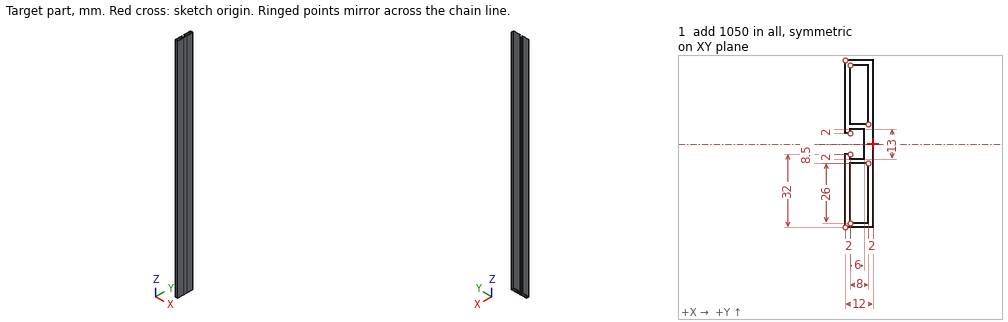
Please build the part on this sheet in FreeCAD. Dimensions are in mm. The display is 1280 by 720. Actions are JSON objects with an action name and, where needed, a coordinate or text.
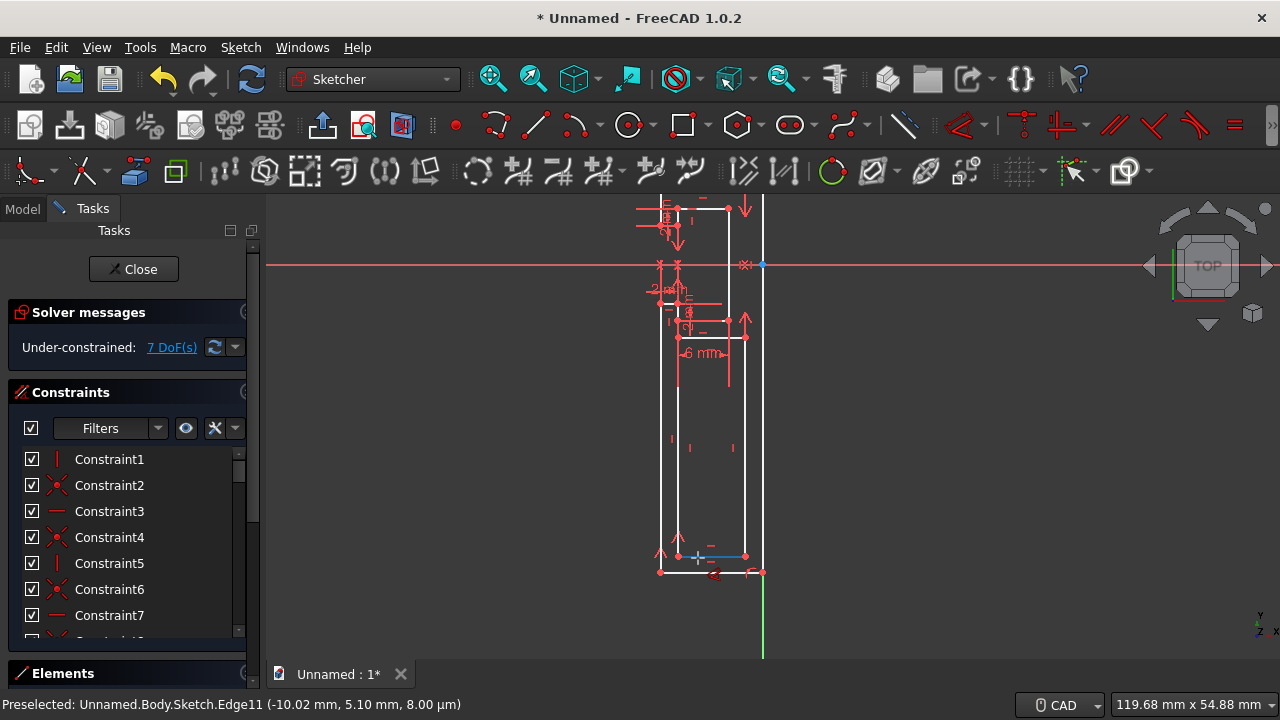
{"action": "left_click", "coordinate": [699, 557]}
{"action": "left_click", "coordinate": [712, 591]}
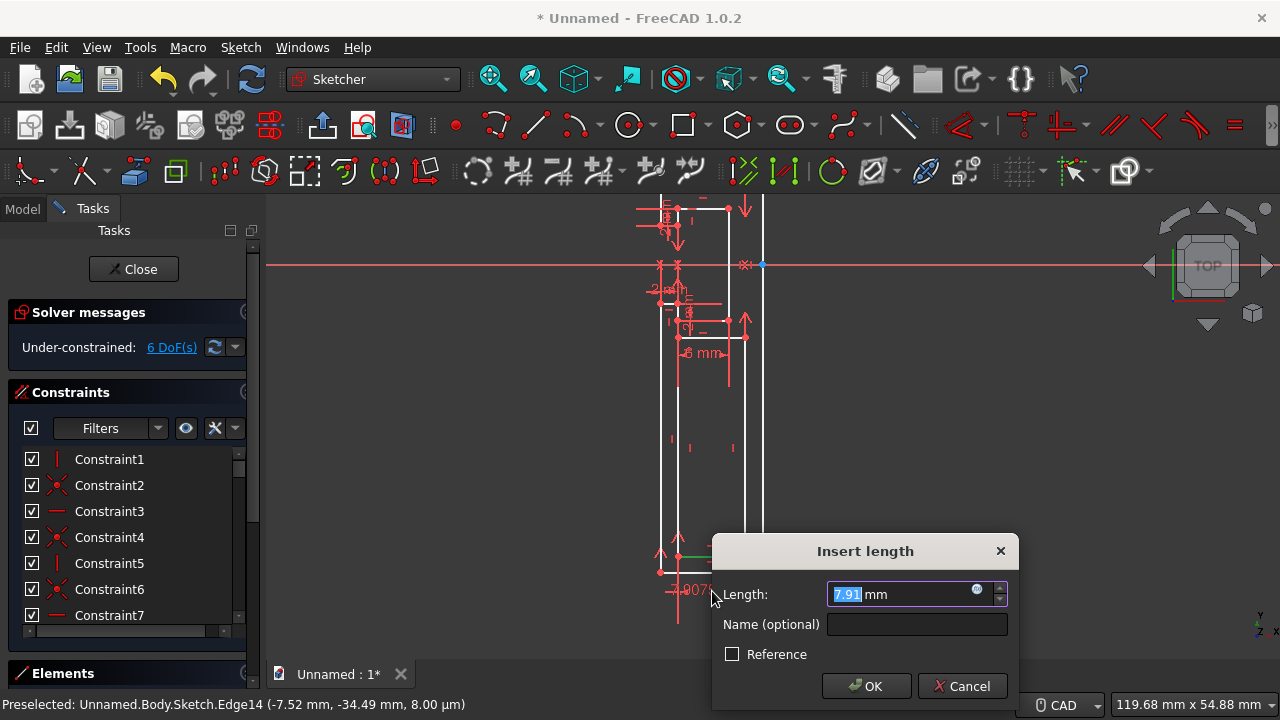
{"action": "type", "text": "8"}
{"action": "key", "text": "Return"}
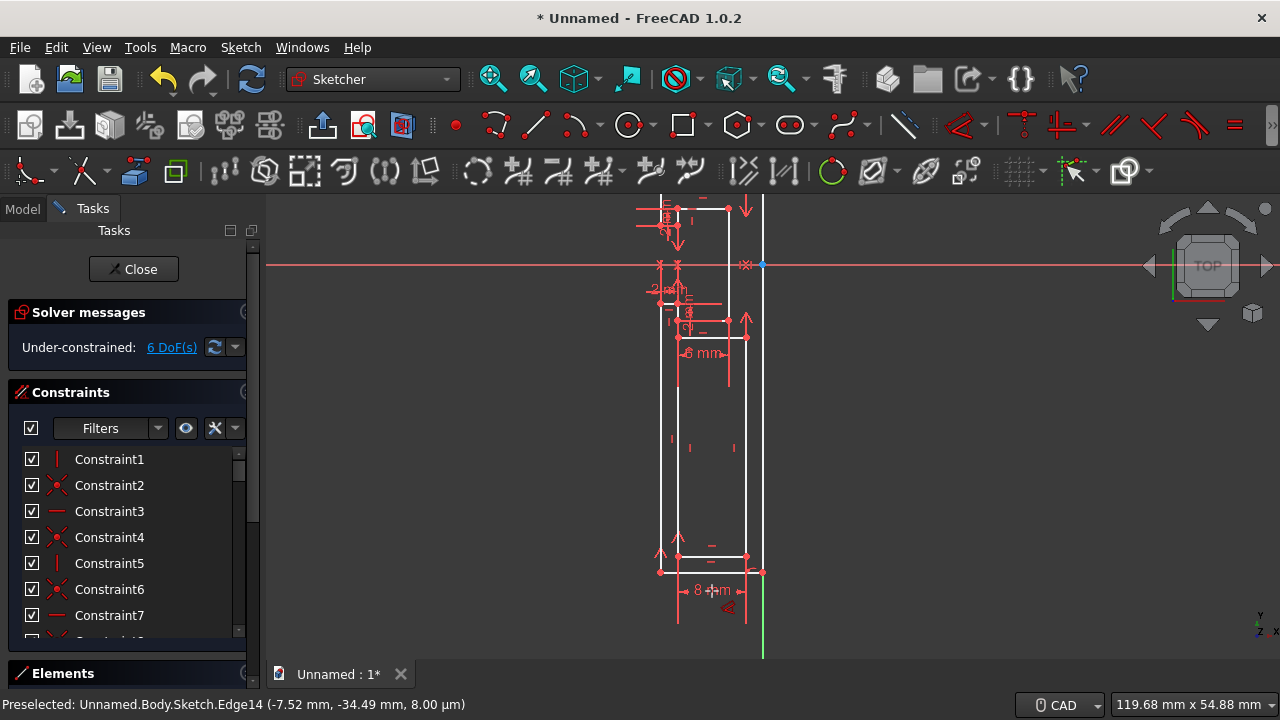
{"action": "left_click", "coordinate": [729, 242]}
{"action": "left_click", "coordinate": [695, 249]}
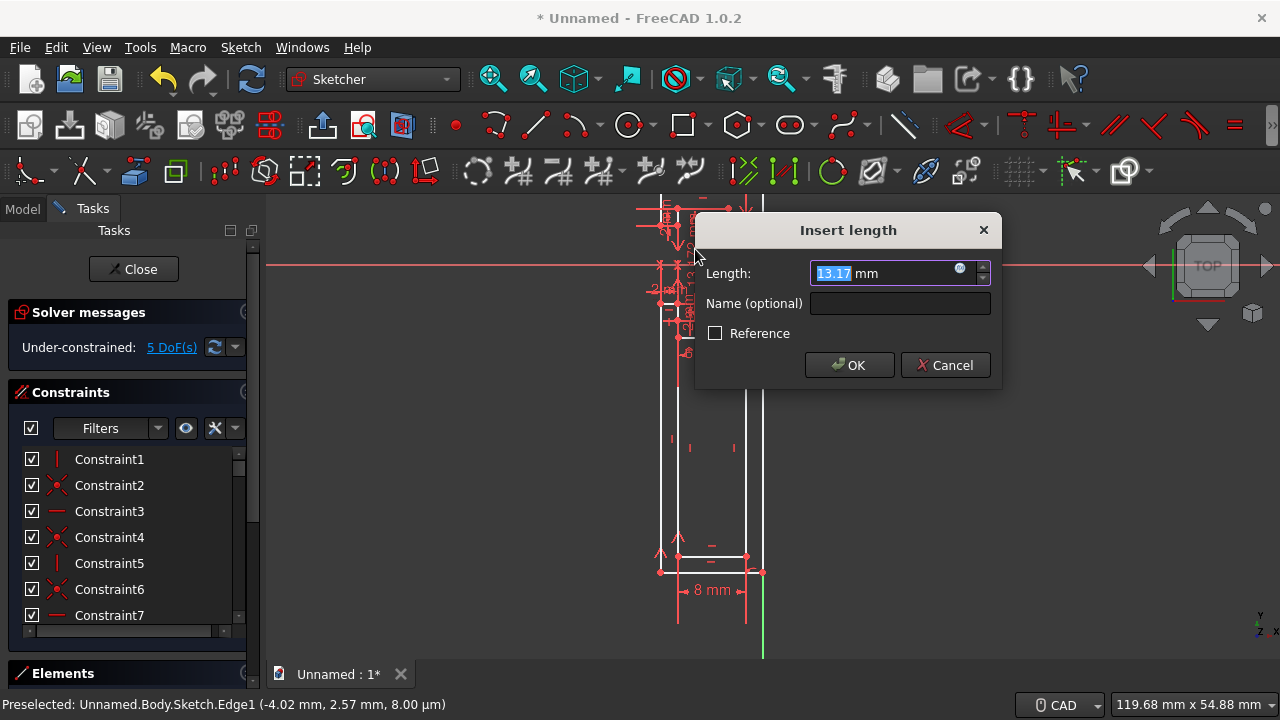
{"action": "type", "text": "13"}
{"action": "key", "text": "Return"}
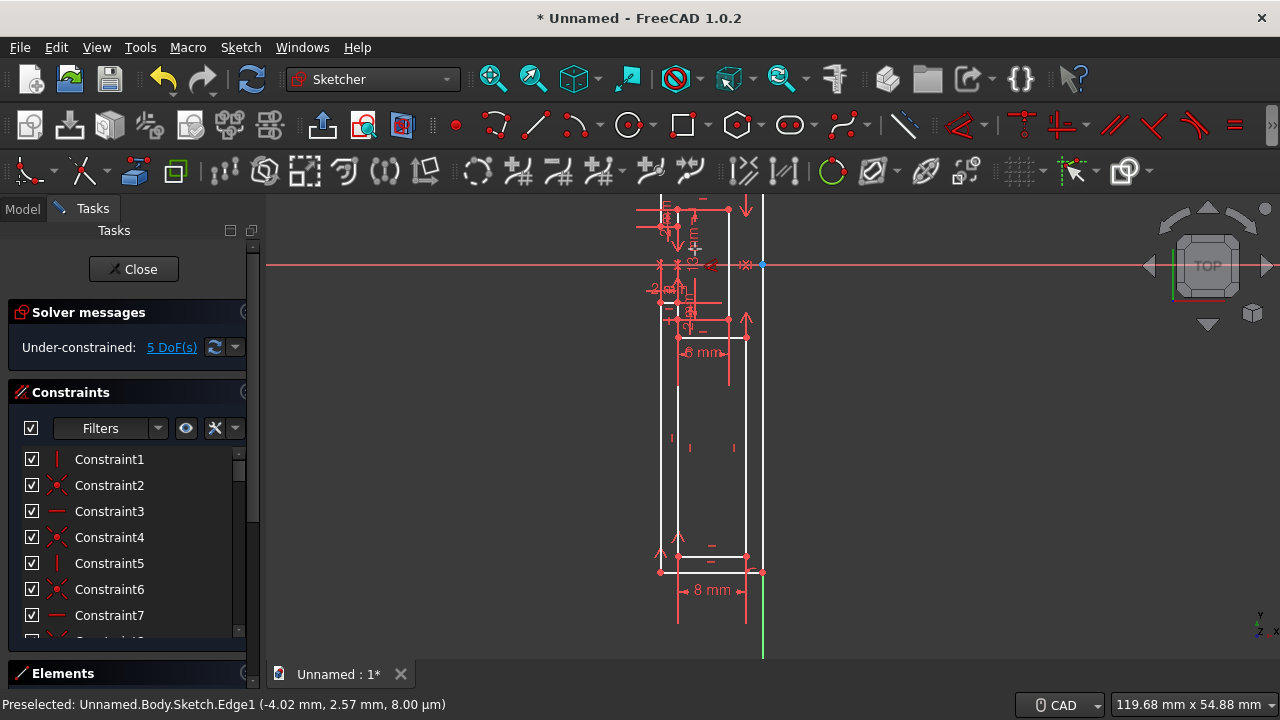
{"action": "left_click", "coordinate": [661, 384]}
{"action": "left_click", "coordinate": [627, 438]}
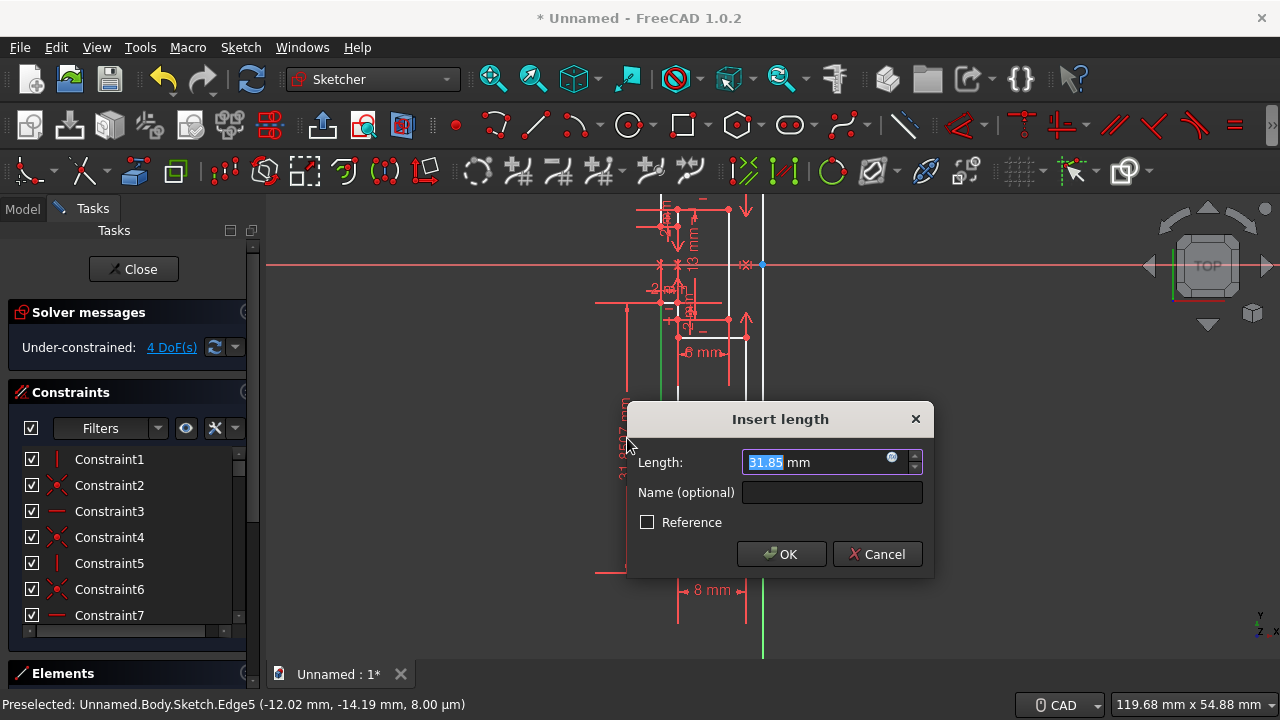
{"action": "type", "text": "32"}
{"action": "key", "text": "Return"}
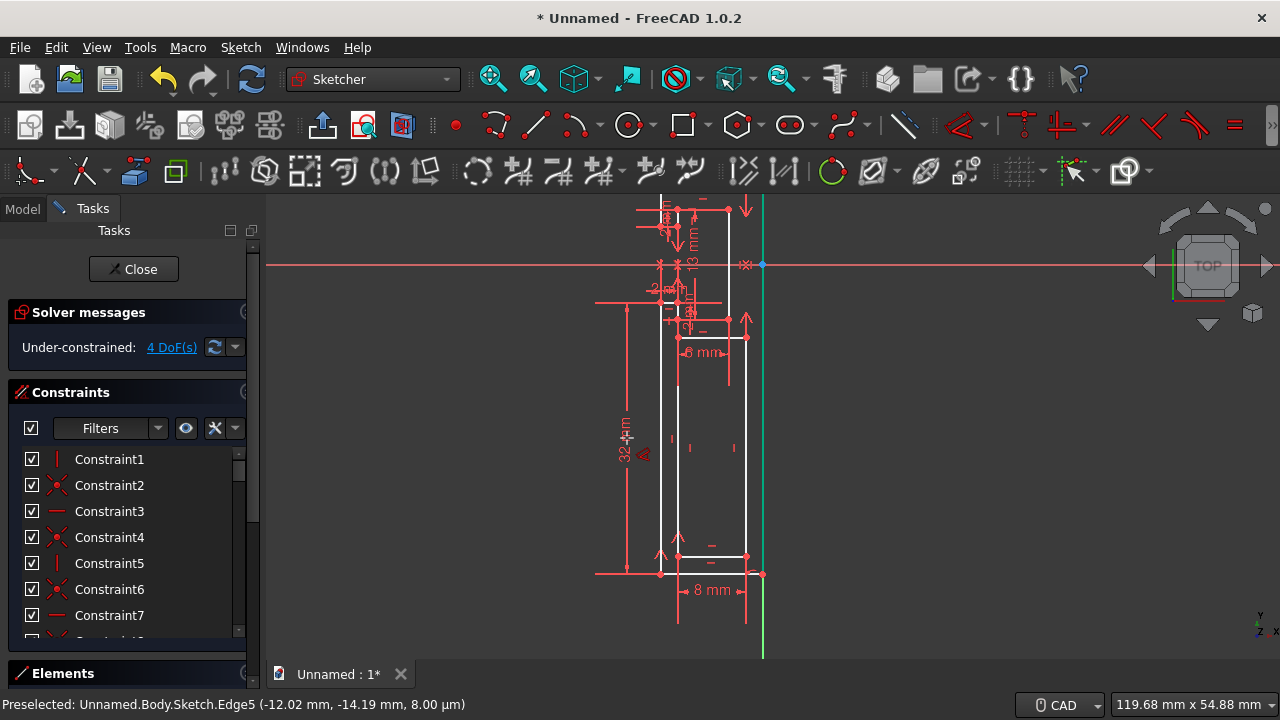
{"action": "left_click", "coordinate": [691, 574]}
{"action": "left_click", "coordinate": [712, 540]}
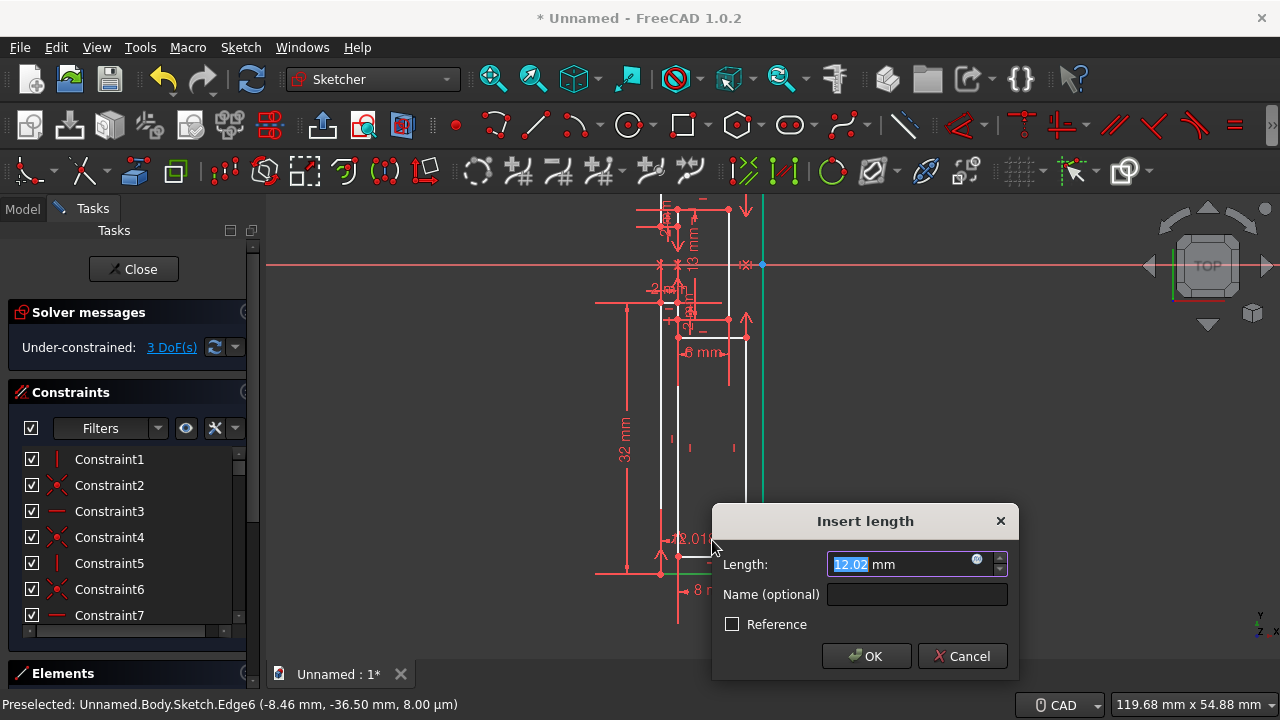
{"action": "type", "text": "12"}
{"action": "key", "text": "Return"}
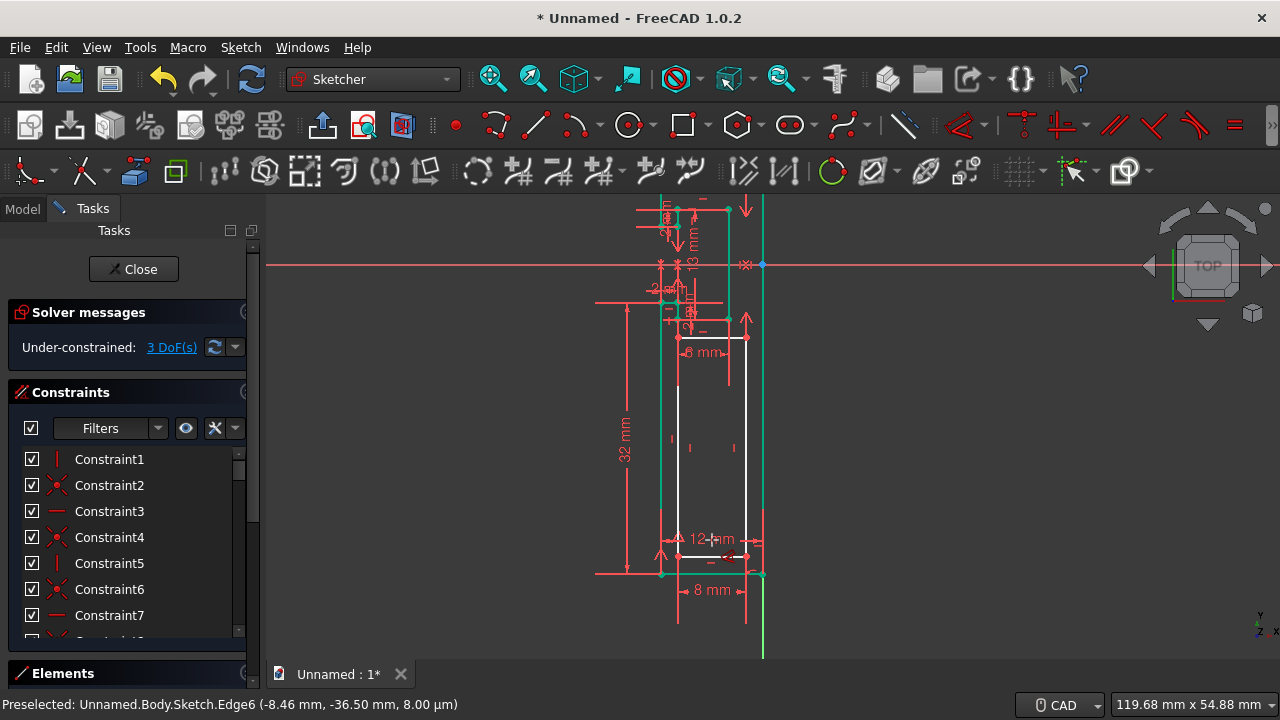
{"action": "left_click", "coordinate": [678, 403]}
{"action": "left_click", "coordinate": [644, 397]}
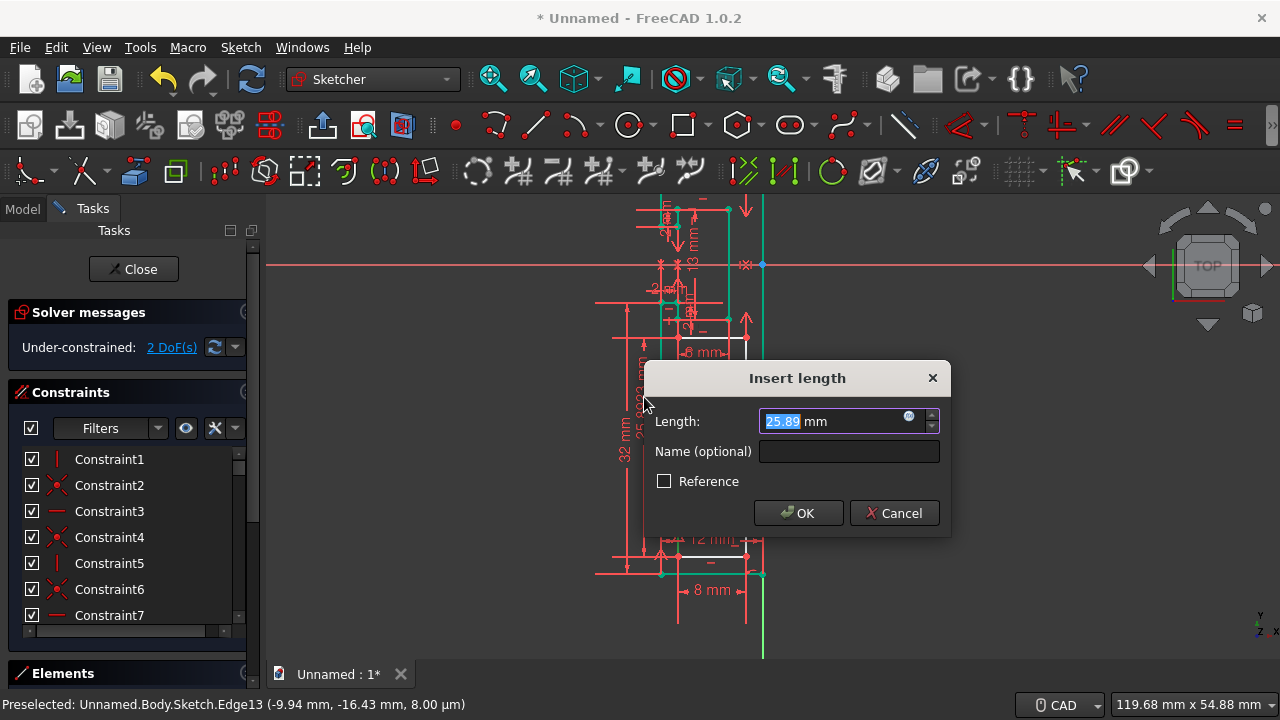
{"action": "type", "text": "26"}
{"action": "key", "text": "Return"}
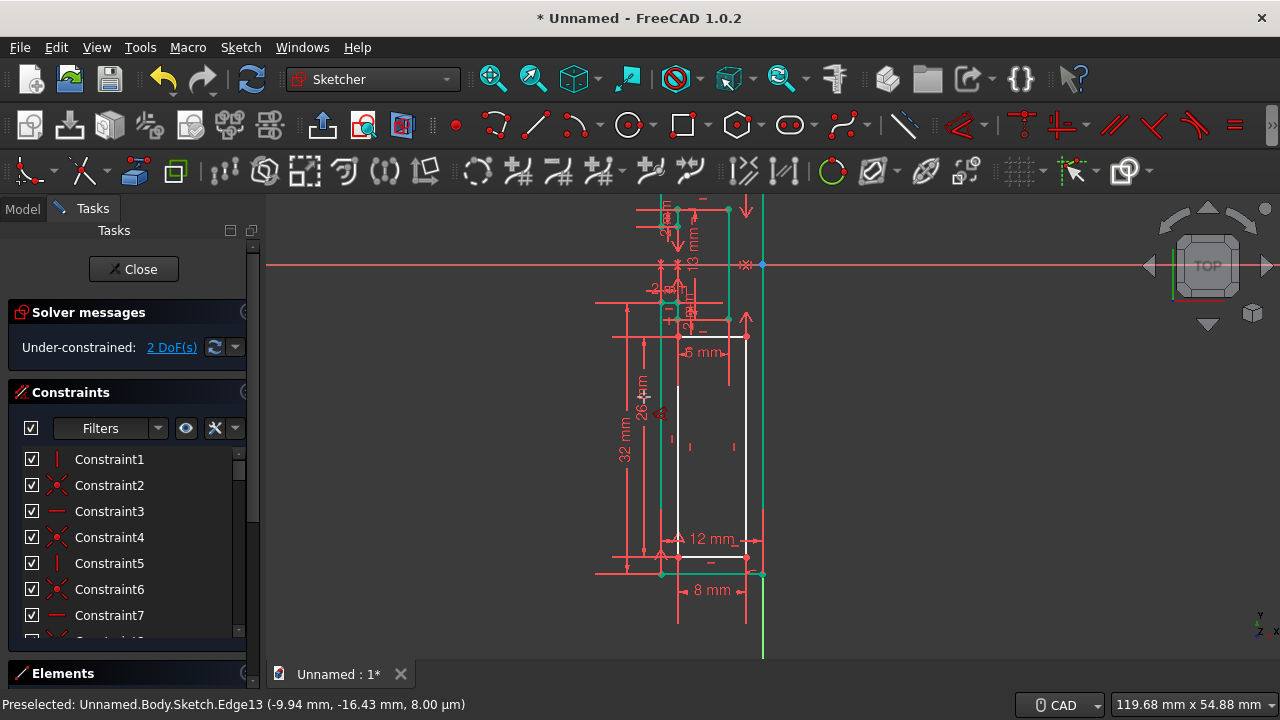
{"action": "scroll", "coordinate": [746, 557], "scroll_direction": "up", "scroll_amount": 5}